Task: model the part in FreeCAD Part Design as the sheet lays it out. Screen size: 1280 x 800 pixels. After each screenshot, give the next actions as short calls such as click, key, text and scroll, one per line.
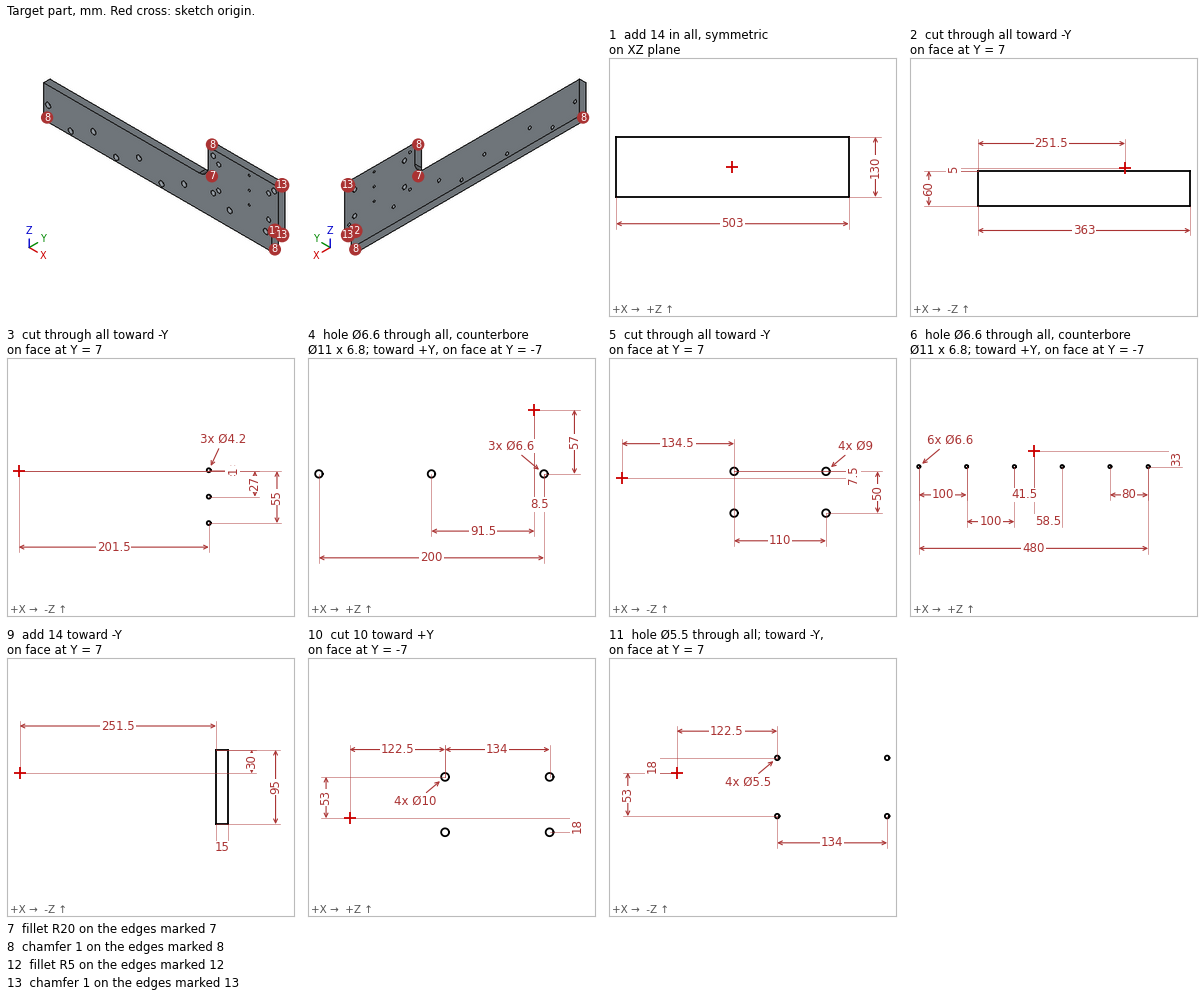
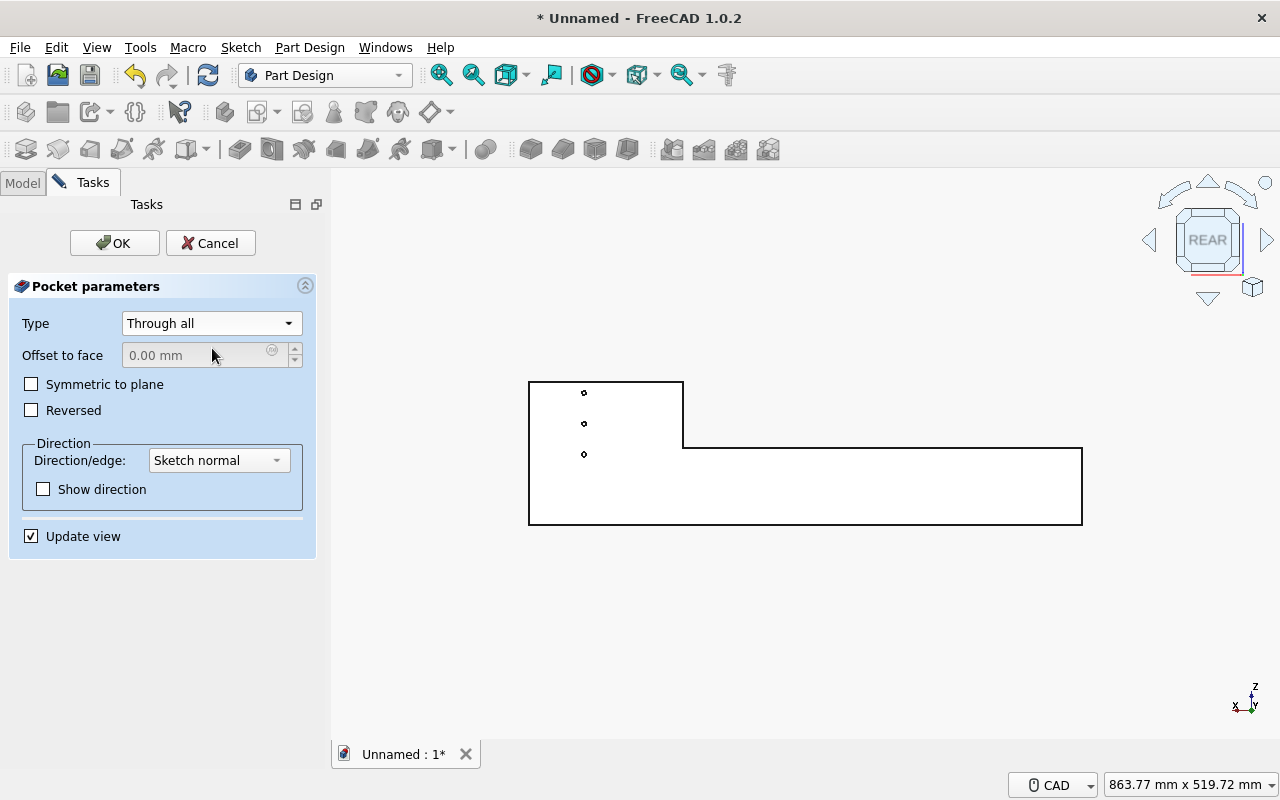
click(115, 243)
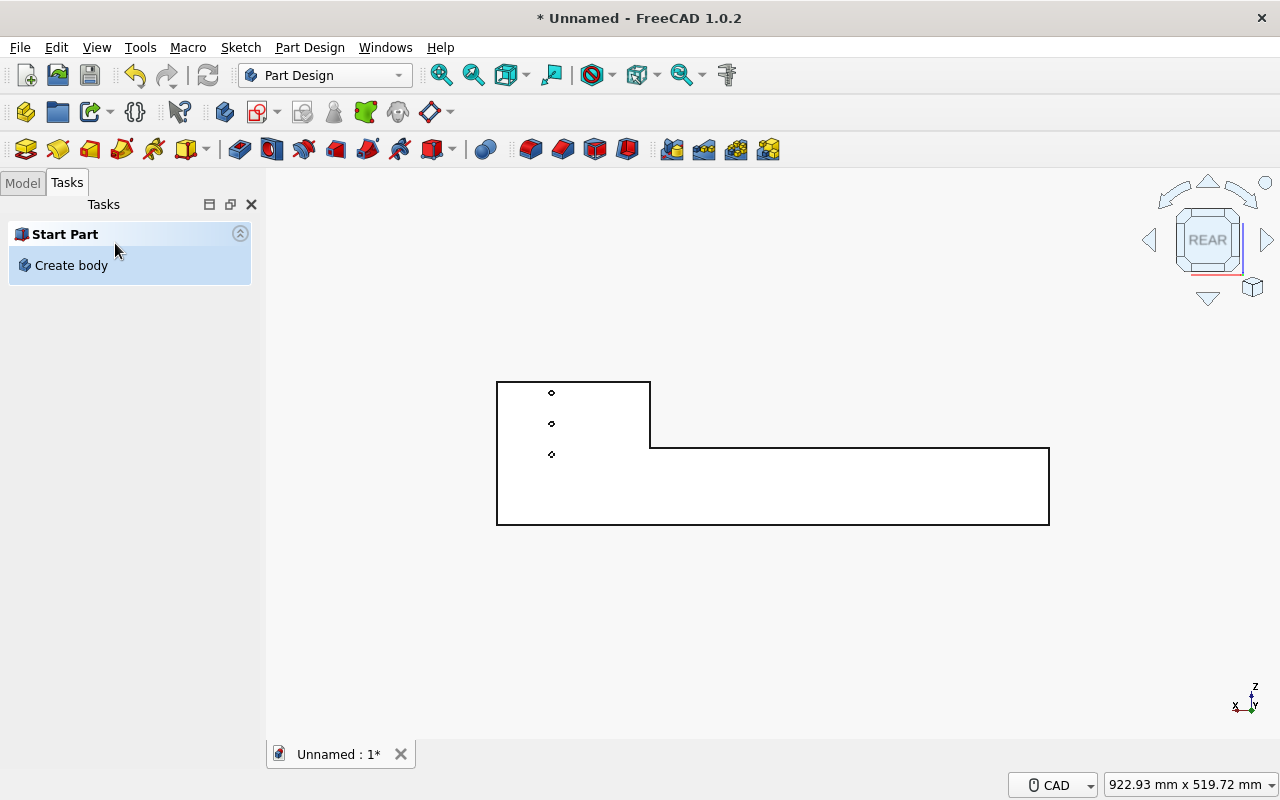
key(0)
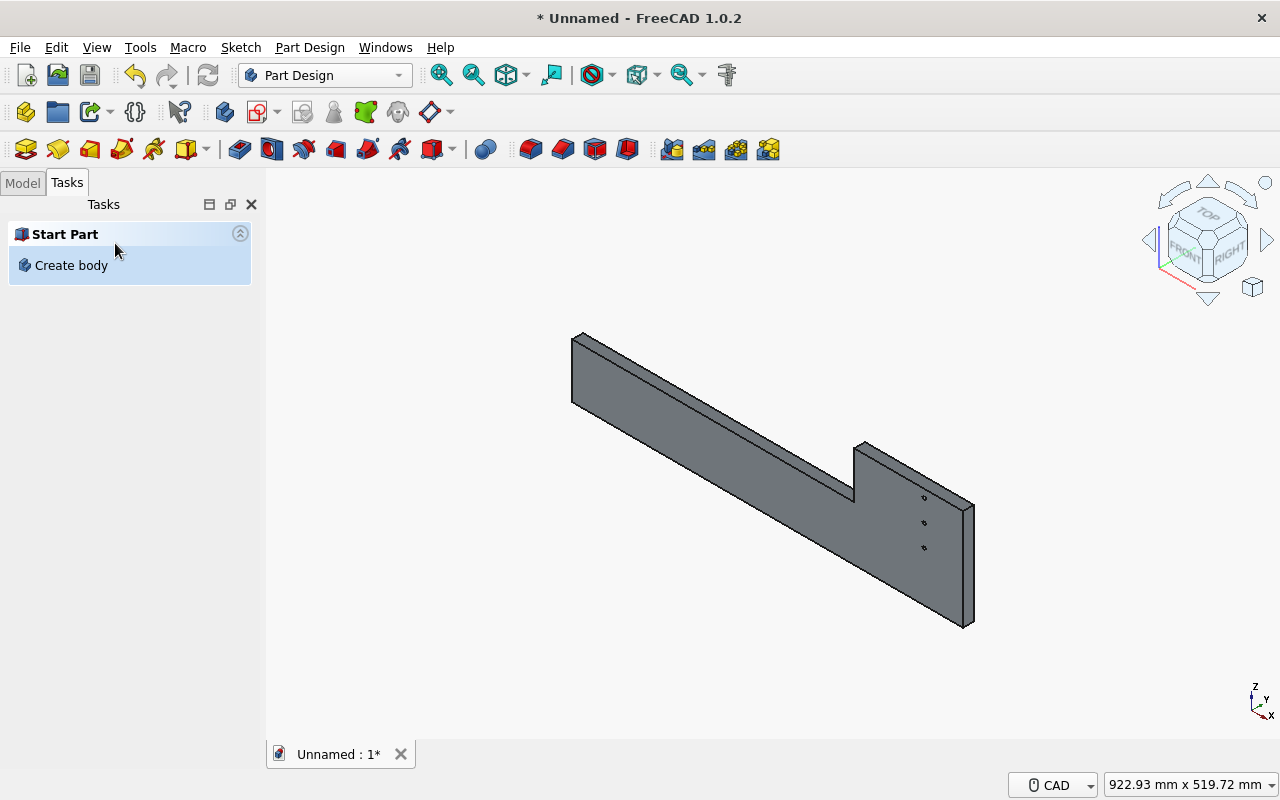
click(879, 537)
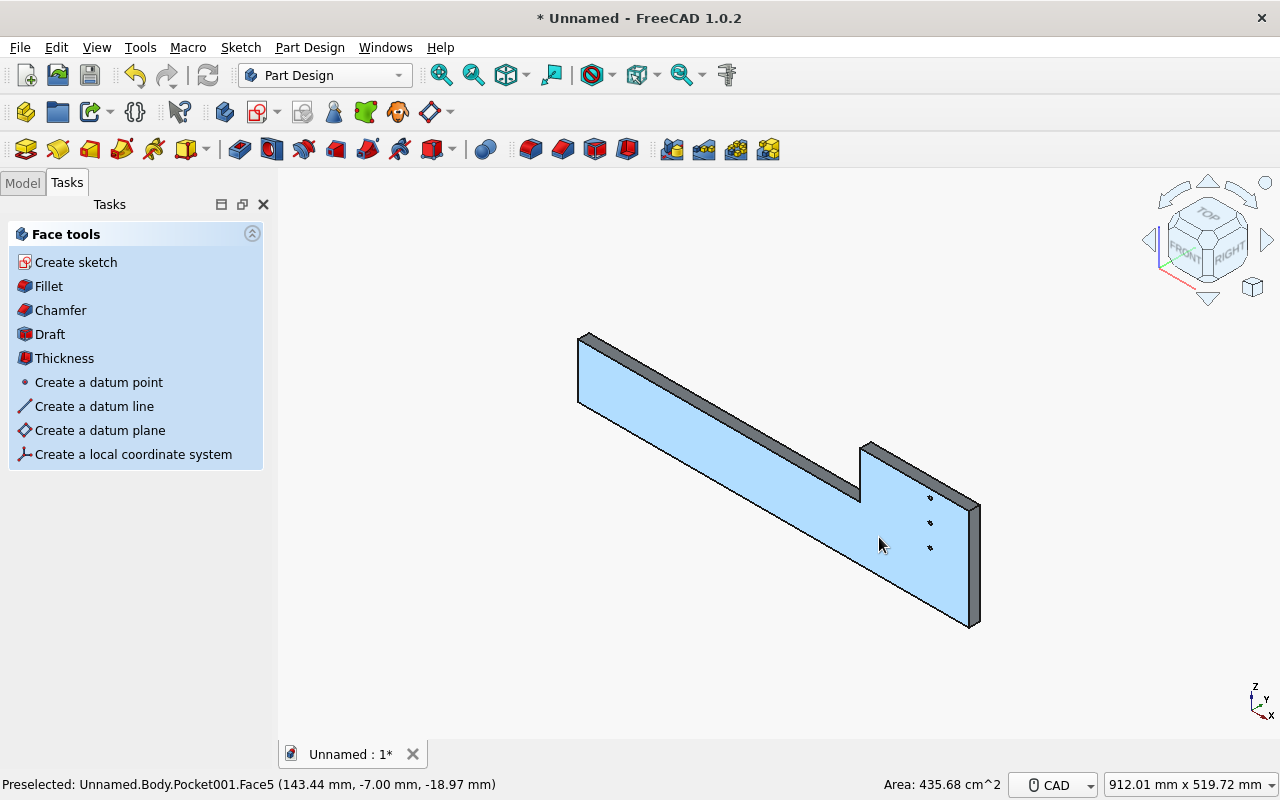
click(258, 112)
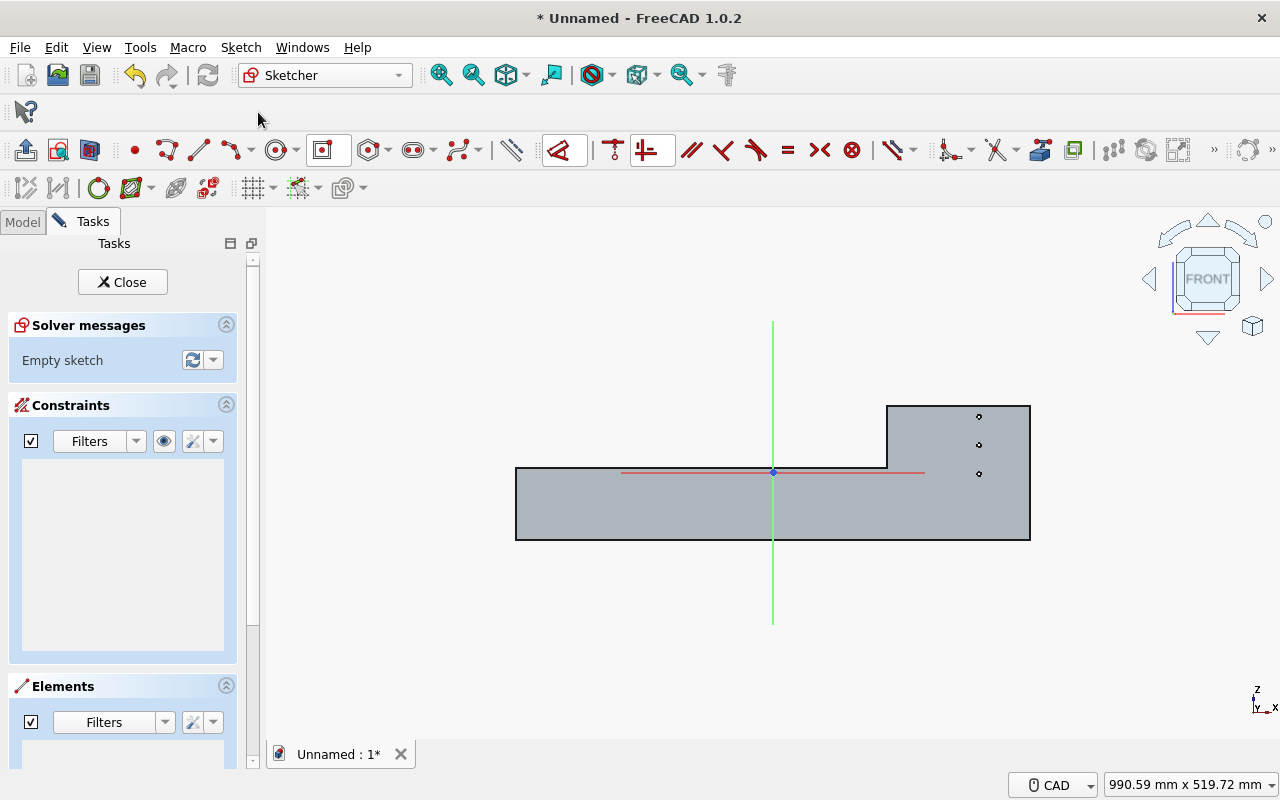
scroll(665, 522, up, 5)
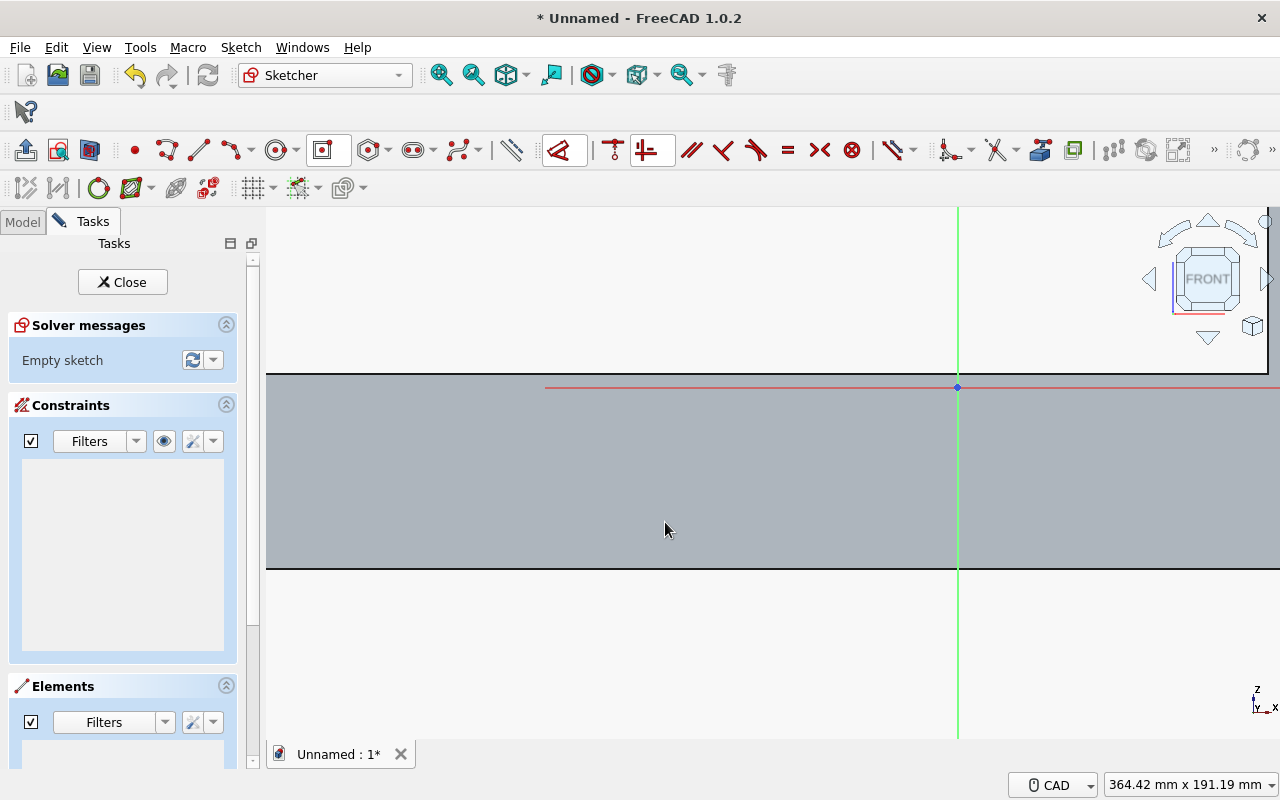
key(g)
key(c)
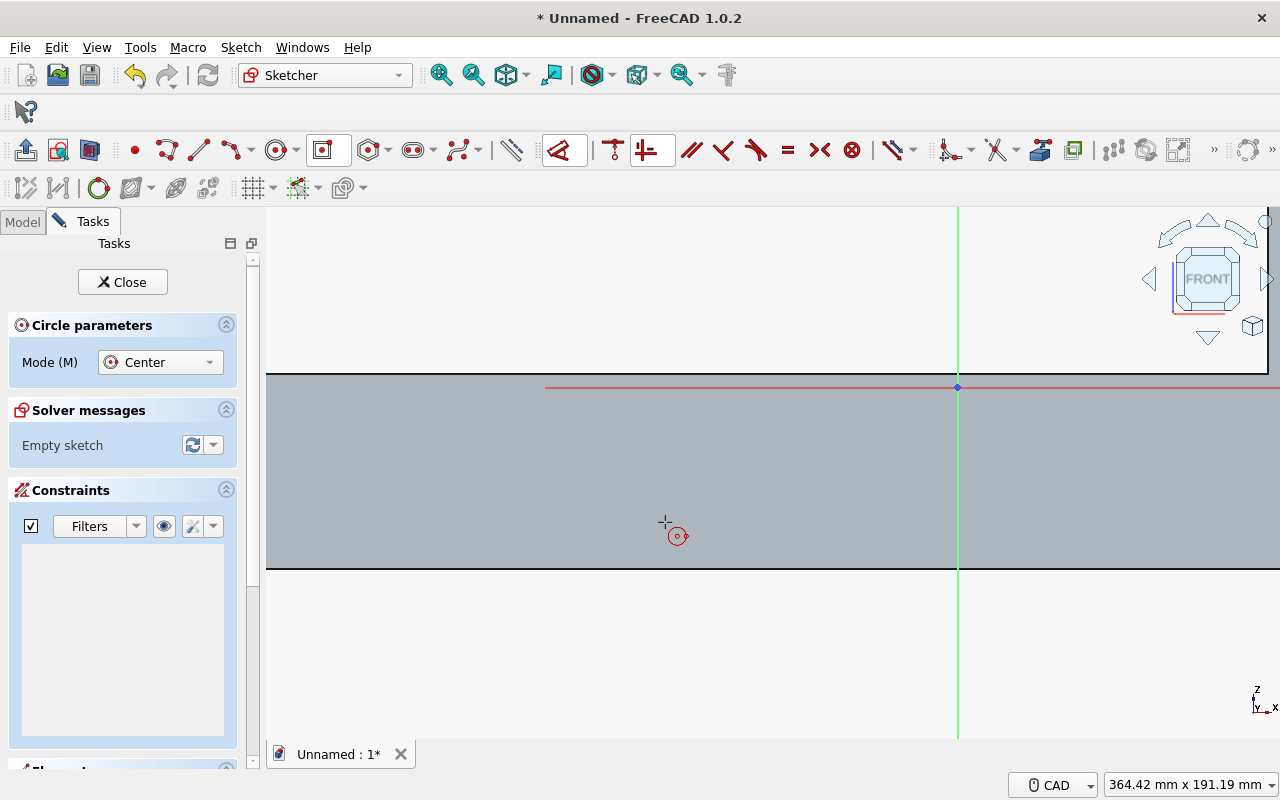
scroll(982, 546, up, 5)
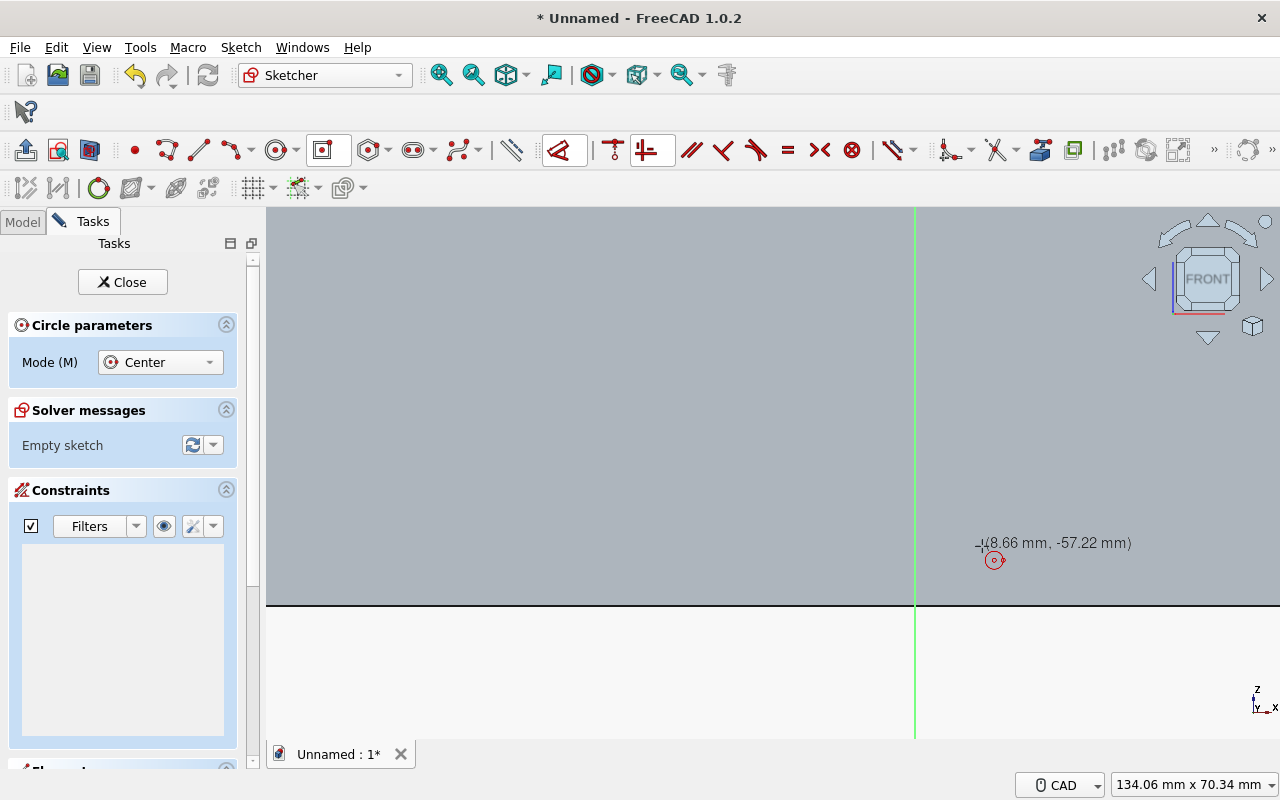
click(980, 546)
click(997, 528)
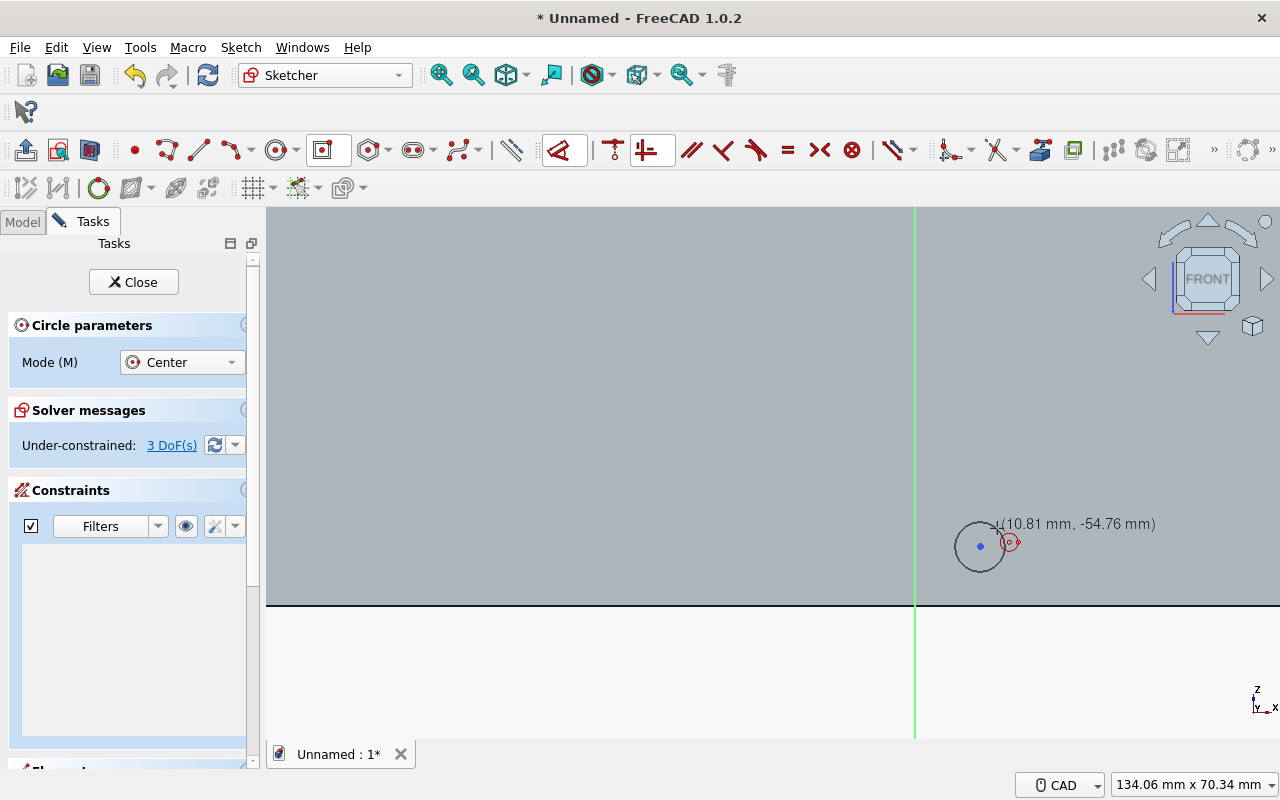
scroll(985, 549, down, 5)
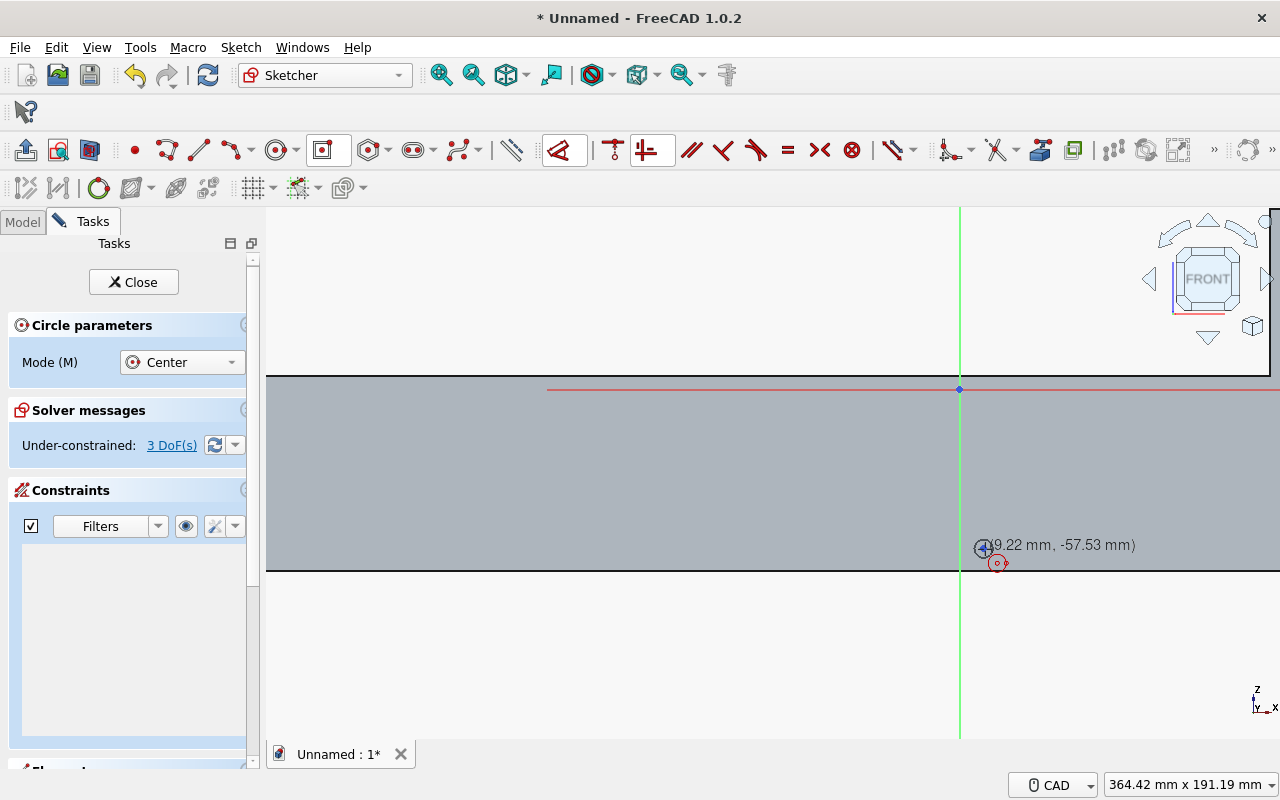
scroll(427, 548, up, 5)